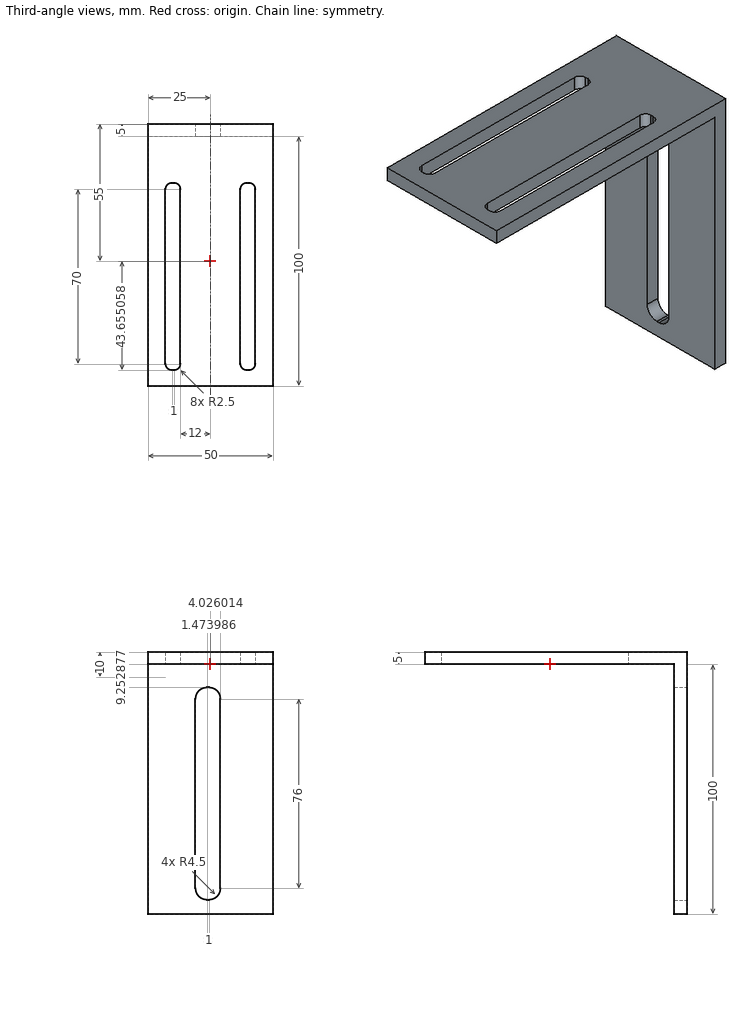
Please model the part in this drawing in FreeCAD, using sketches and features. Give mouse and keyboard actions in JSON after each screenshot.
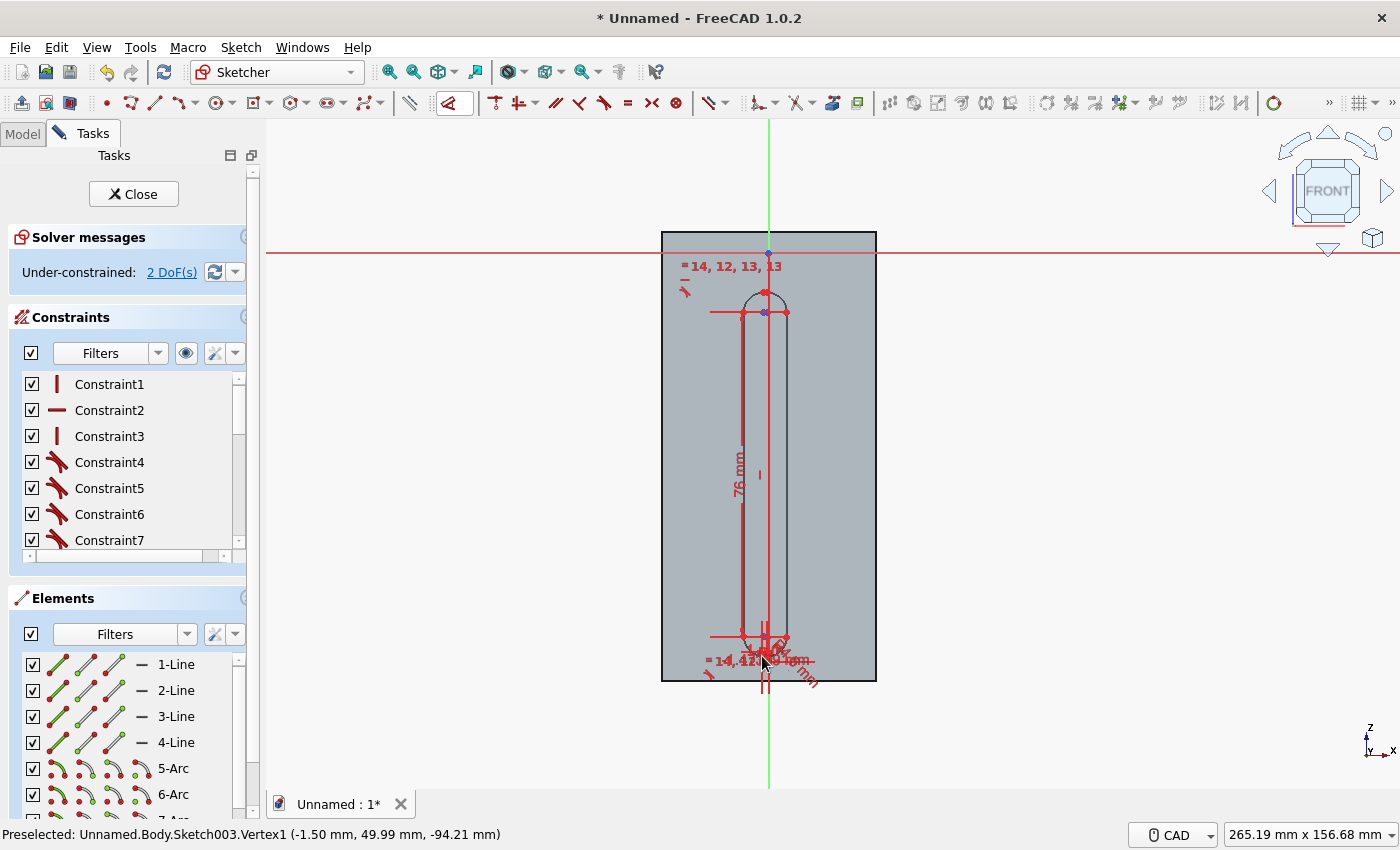
{"action": "scroll", "coordinate": [787, 637], "scroll_direction": "up", "scroll_amount": 5}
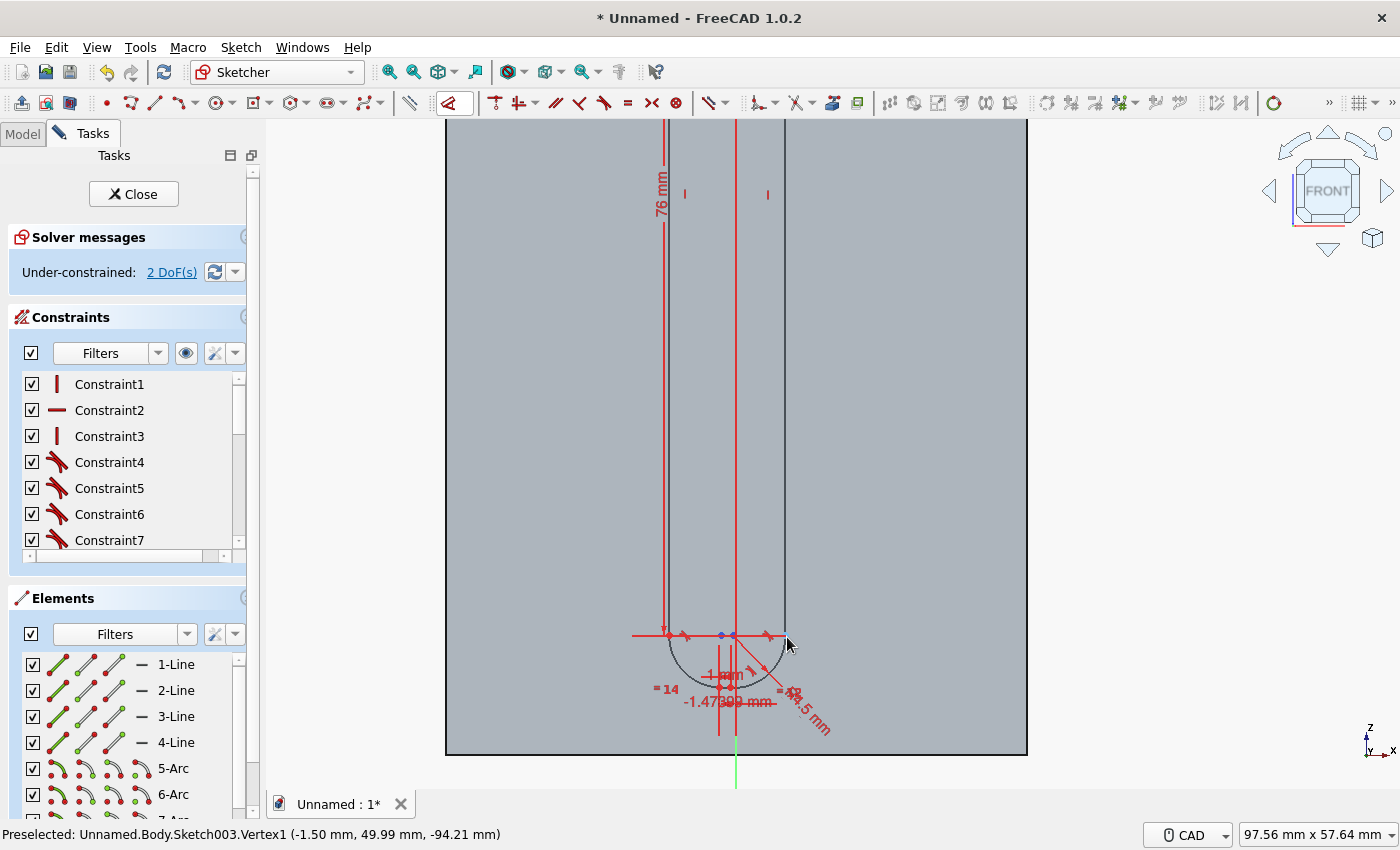
{"action": "left_click", "coordinate": [785, 636]}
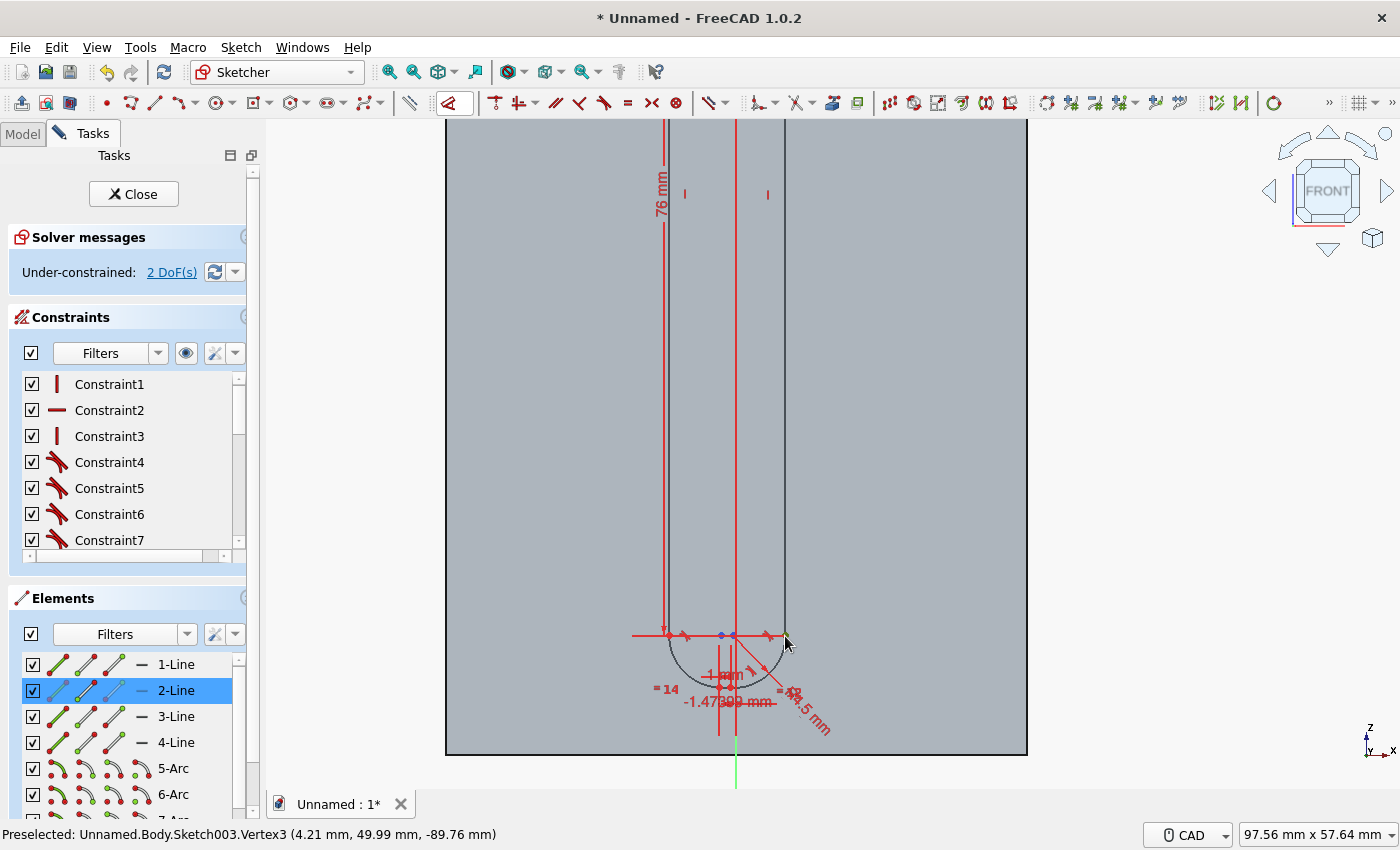
{"action": "left_click", "coordinate": [468, 104]}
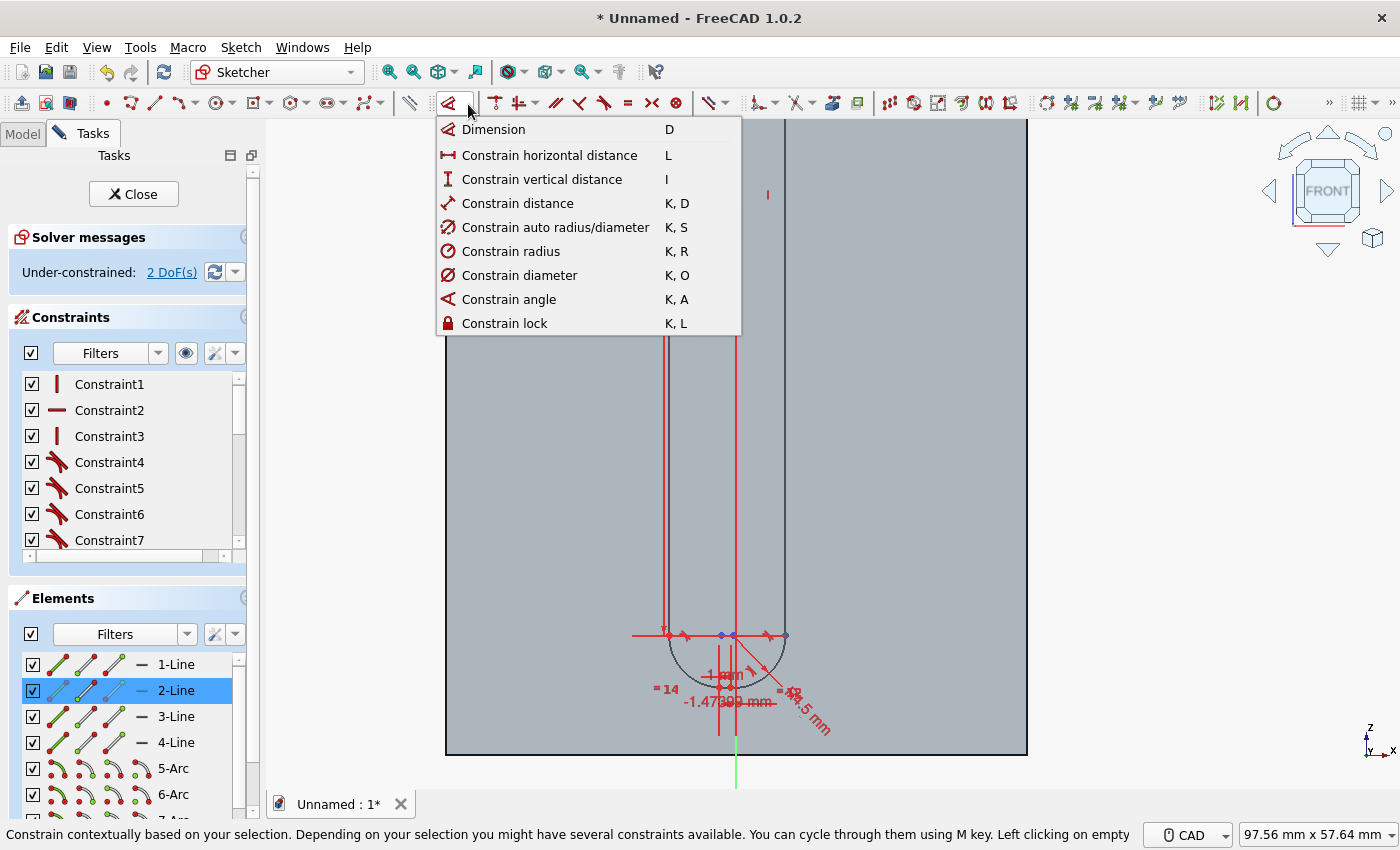
{"action": "left_click", "coordinate": [589, 155]}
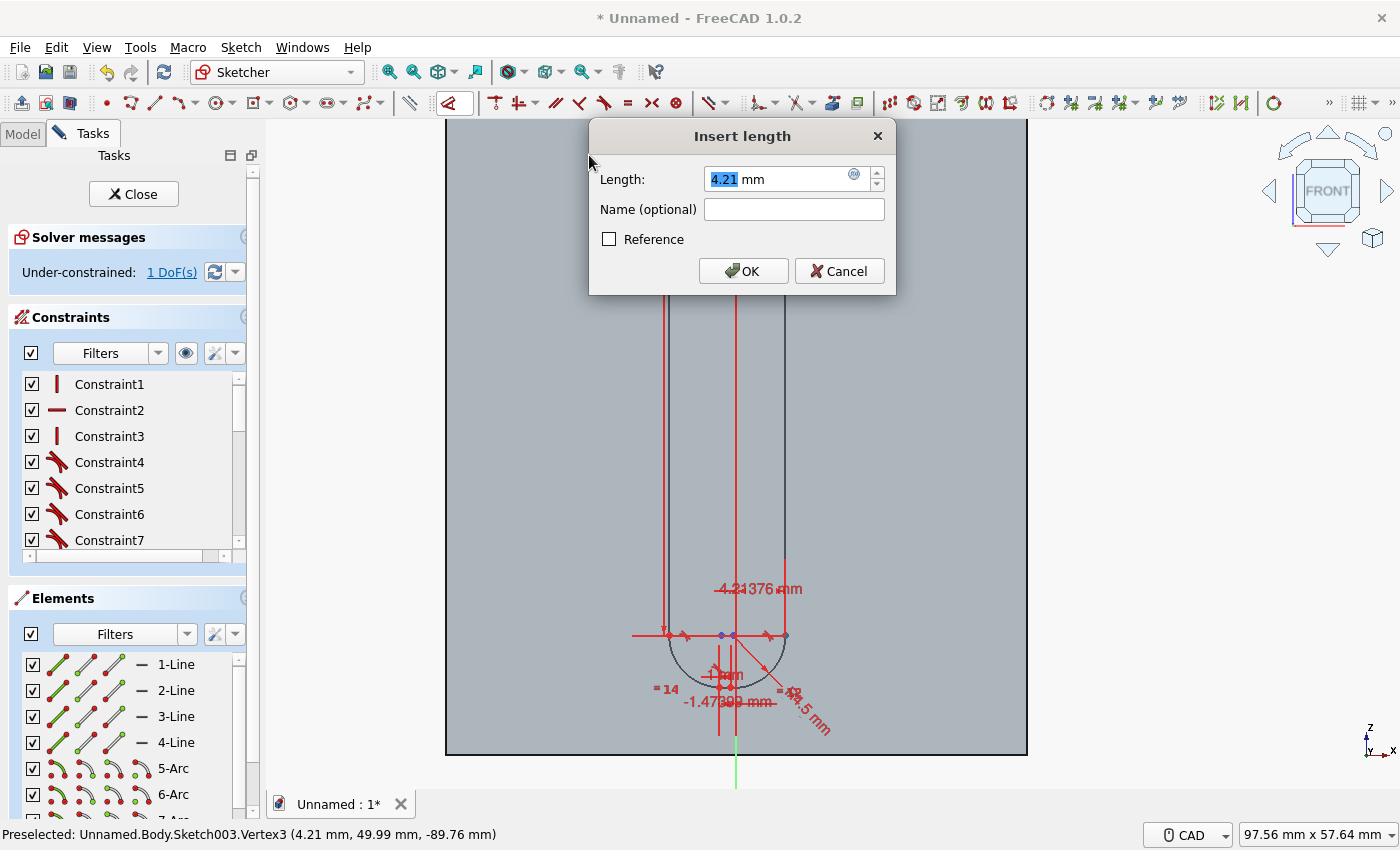
{"action": "type", "text": "4.026014"}
{"action": "key", "text": "Return"}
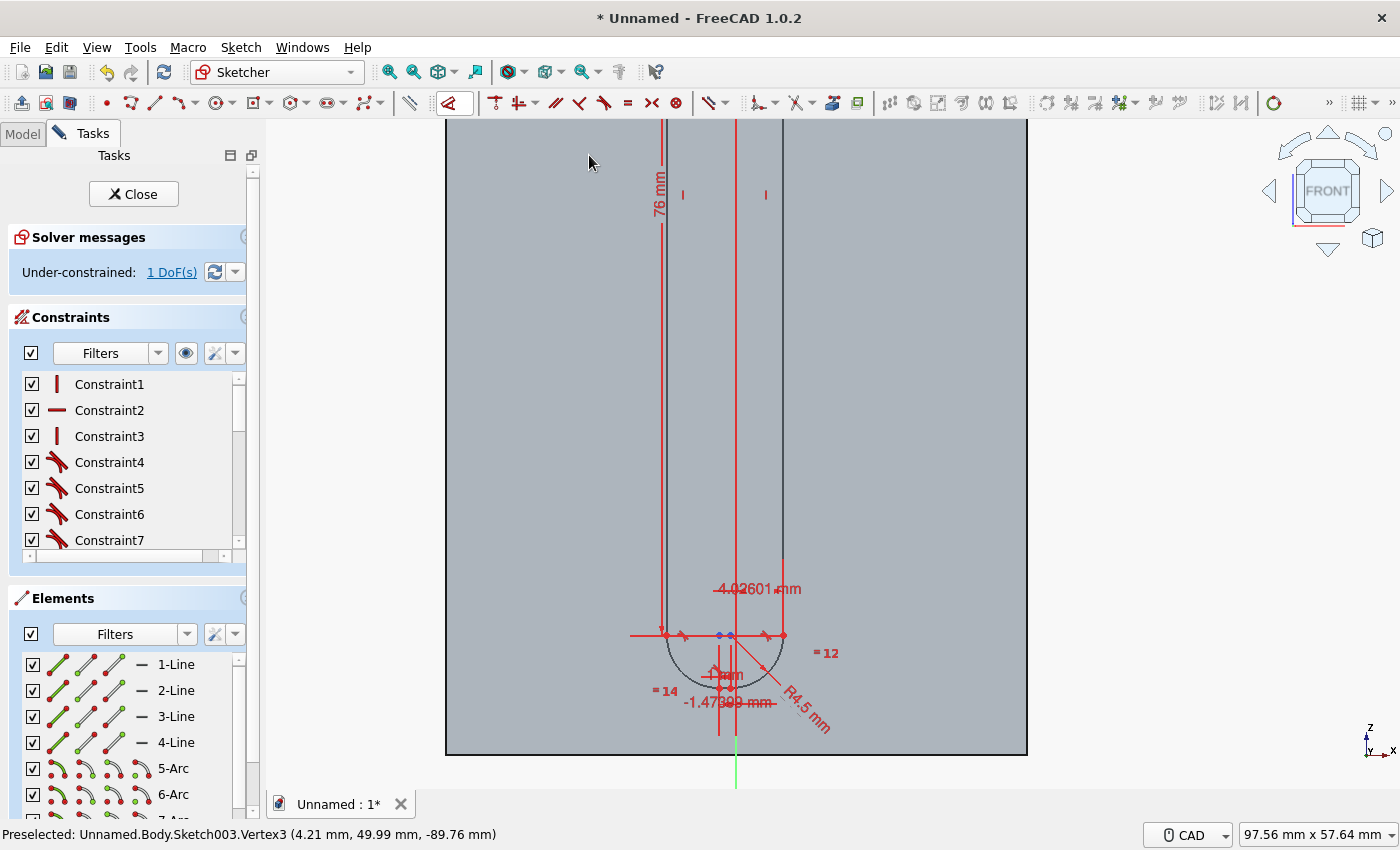
{"action": "scroll", "coordinate": [787, 637], "scroll_direction": "down", "scroll_amount": 5}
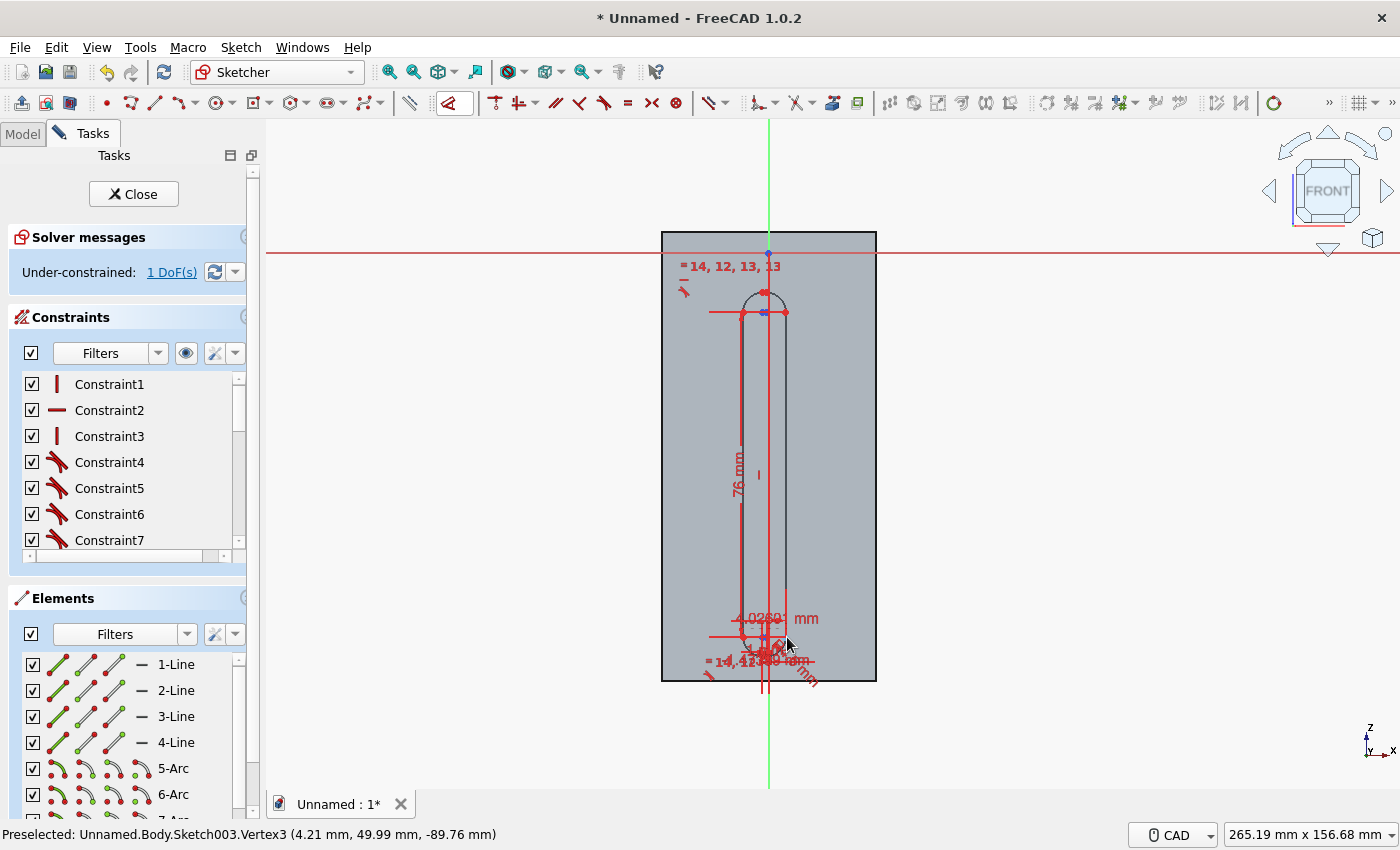
{"action": "scroll", "coordinate": [767, 293], "scroll_direction": "up", "scroll_amount": 6}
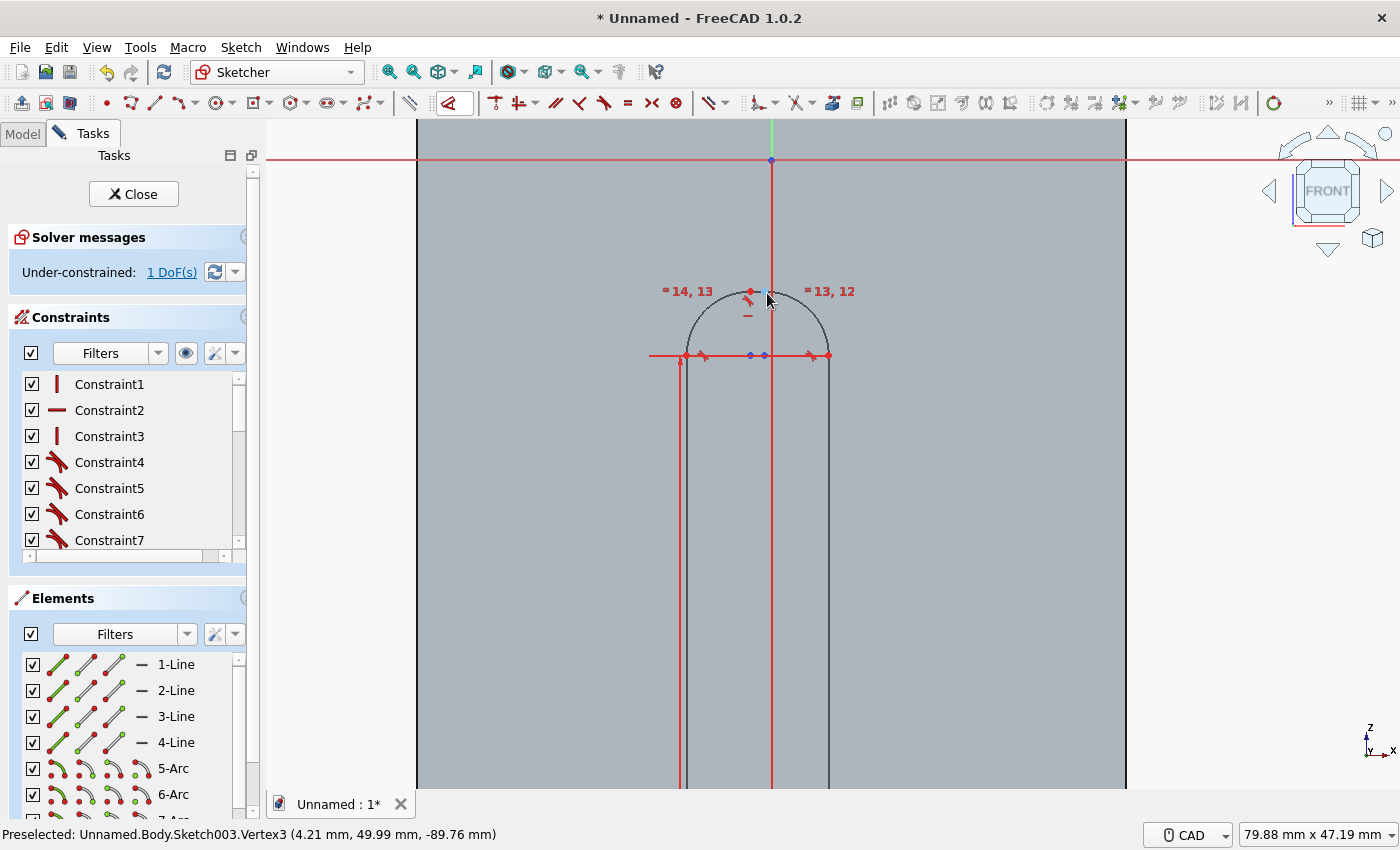
{"action": "left_click", "coordinate": [765, 292]}